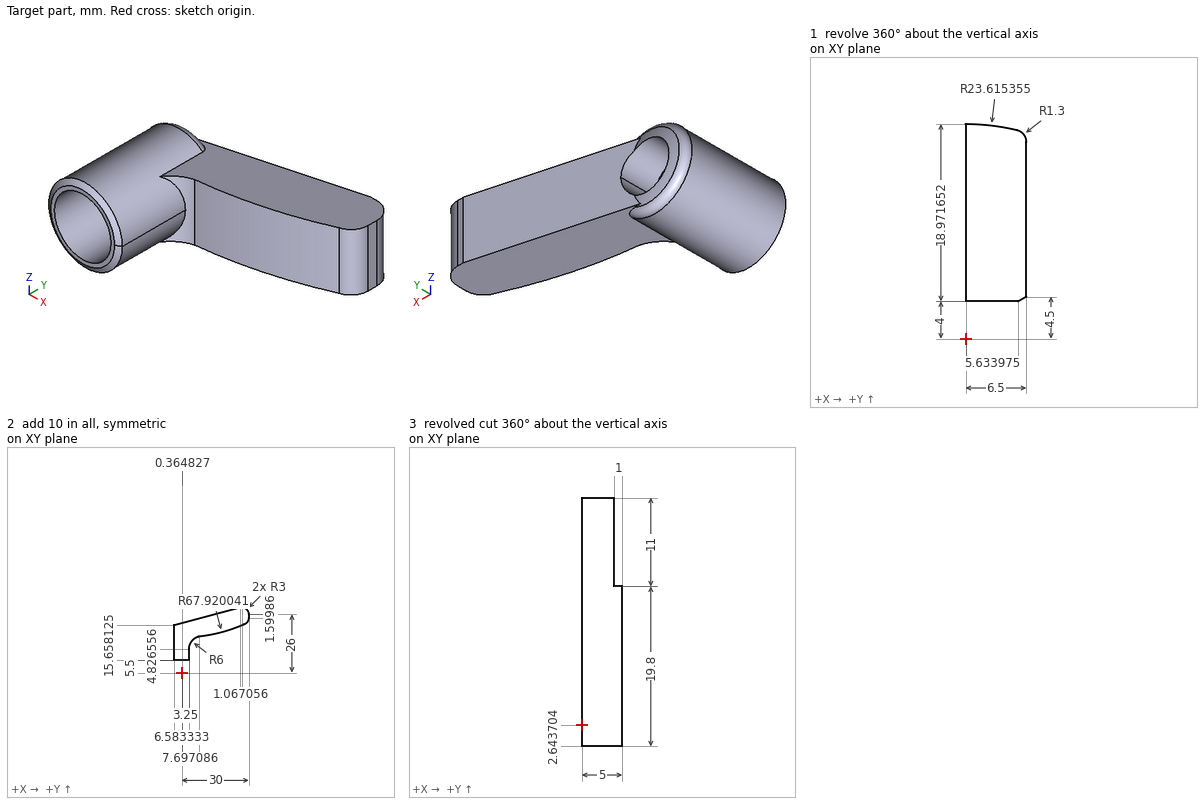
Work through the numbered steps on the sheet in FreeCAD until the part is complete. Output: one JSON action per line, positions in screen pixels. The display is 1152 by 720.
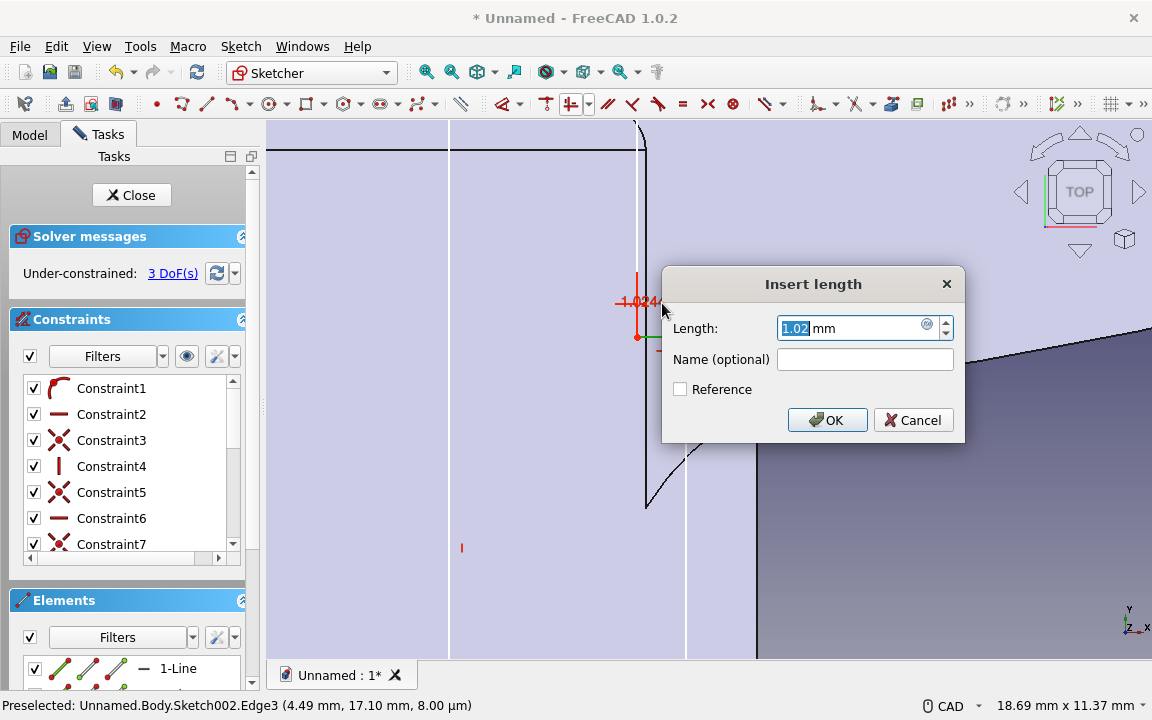
{"action": "type", "text": "1"}
{"action": "key", "text": "Return"}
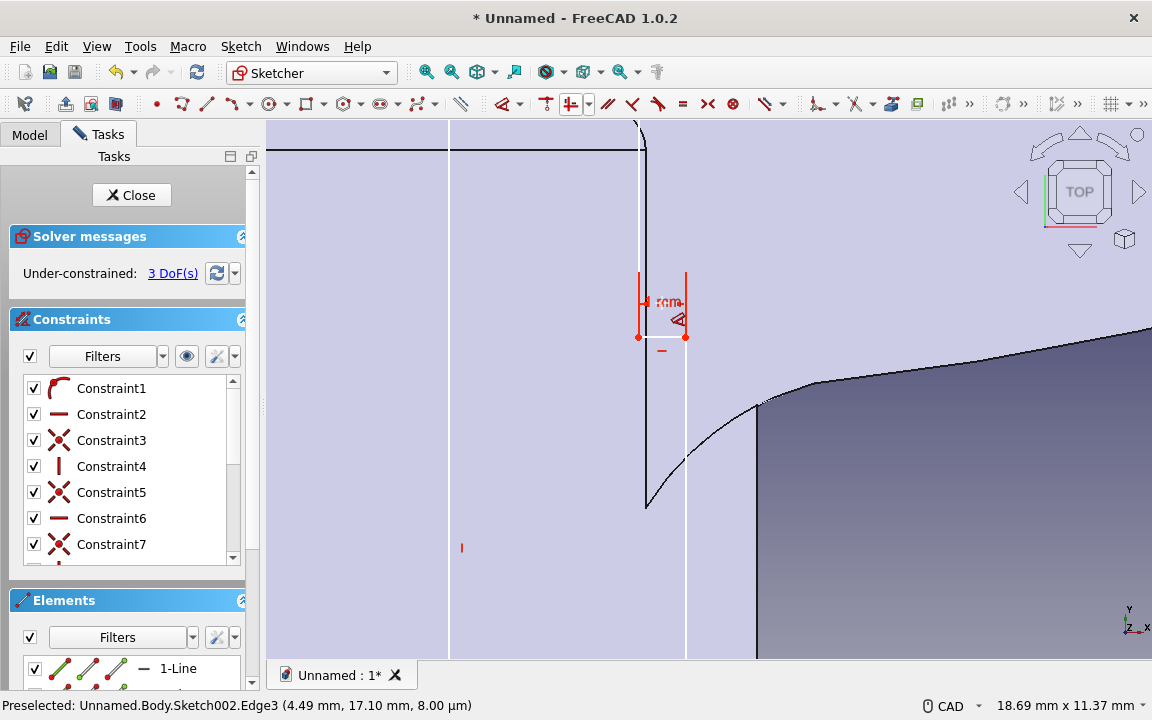
{"action": "scroll", "coordinate": [664, 339], "scroll_direction": "down", "scroll_amount": 7}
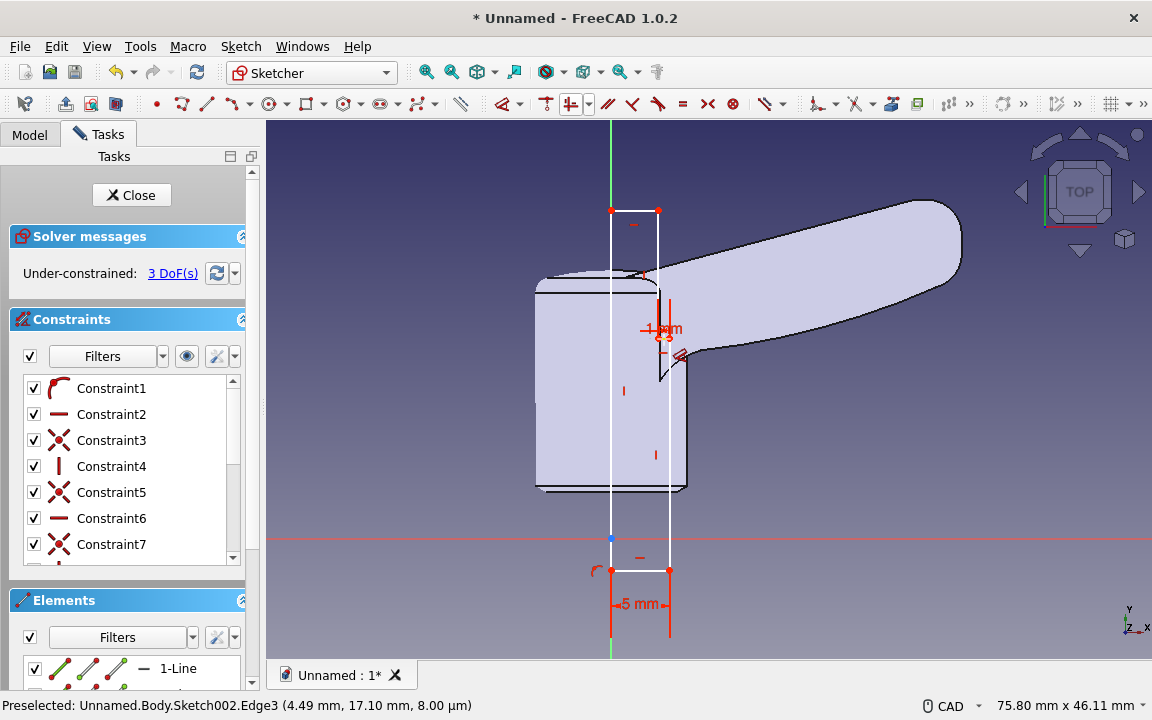
{"action": "left_click", "coordinate": [658, 300]}
{"action": "left_click", "coordinate": [692, 275]}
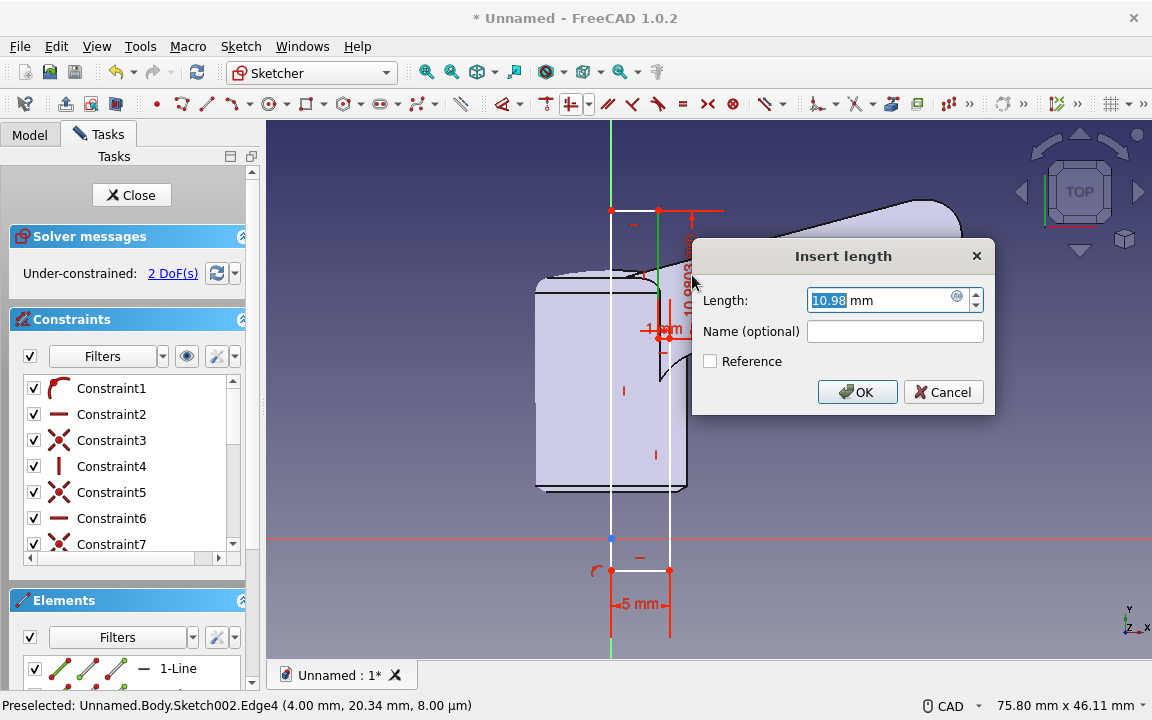
{"action": "type", "text": "11"}
{"action": "key", "text": "Return"}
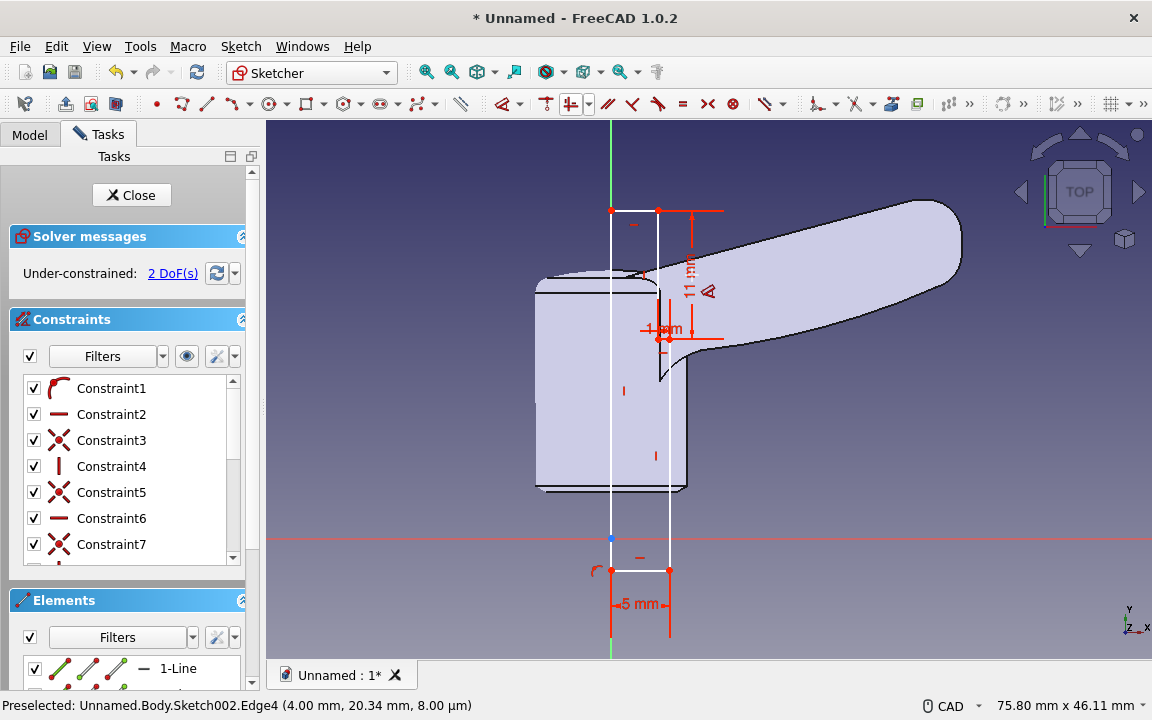
{"action": "left_click", "coordinate": [670, 501]}
{"action": "left_click", "coordinate": [704, 455]}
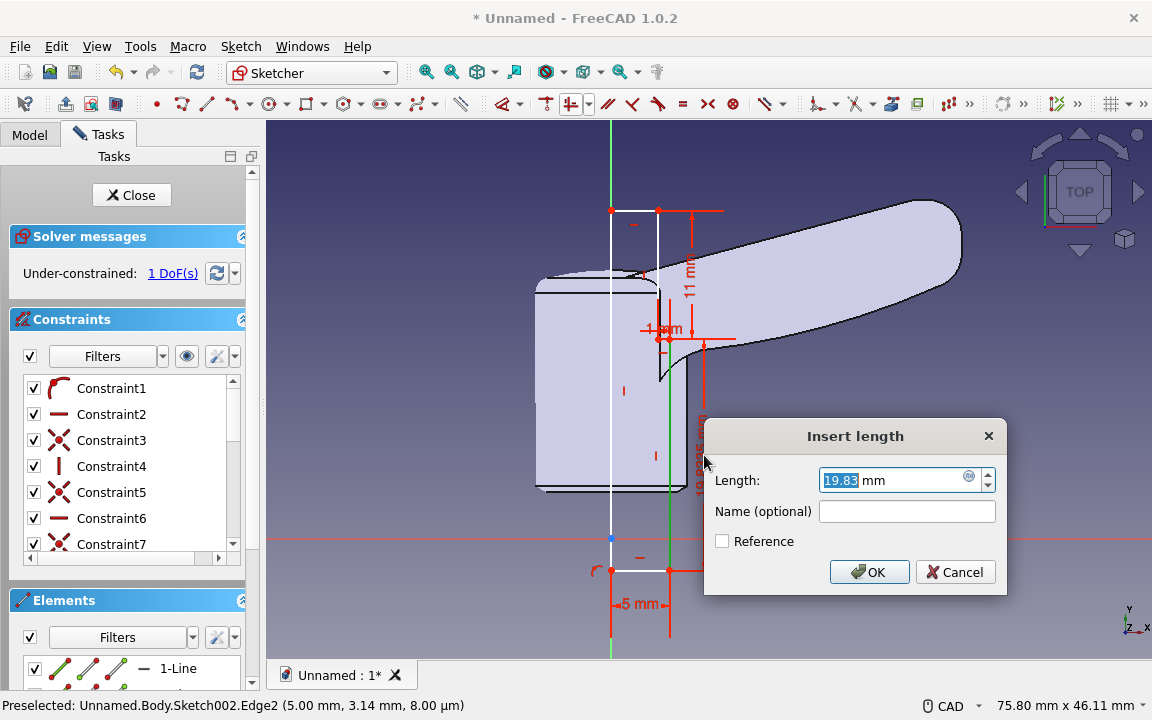
{"action": "type", "text": "19.8"}
{"action": "key", "text": "Return"}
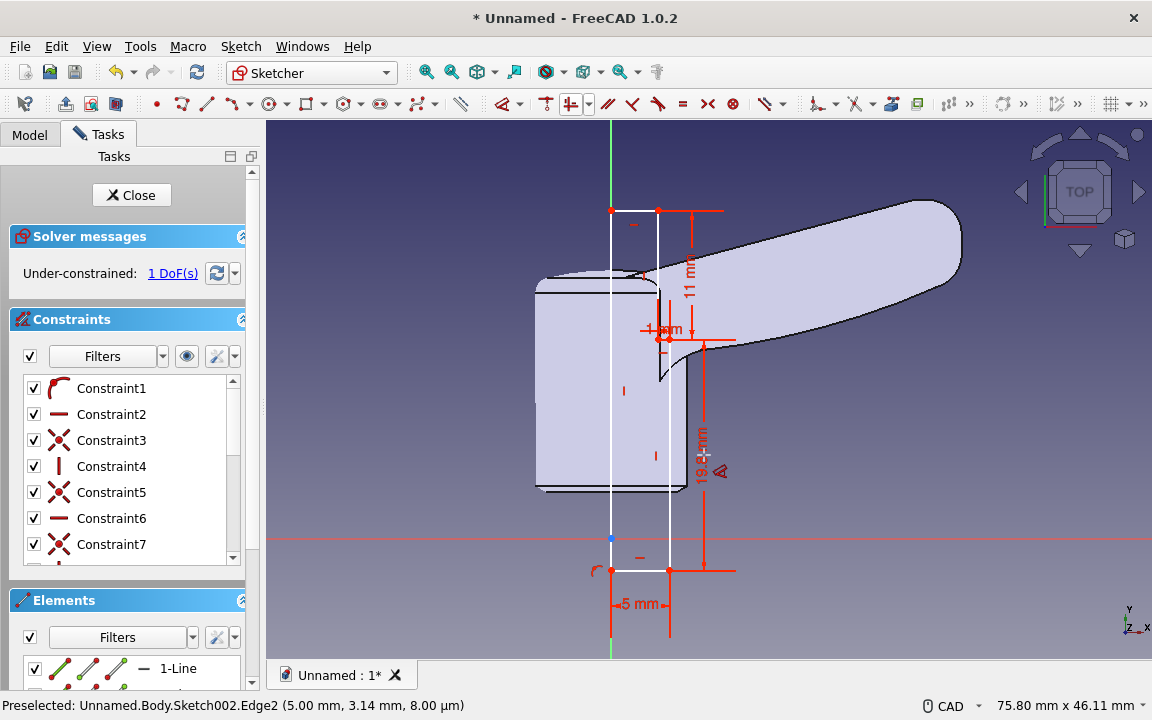
{"action": "scroll", "coordinate": [611, 571], "scroll_direction": "up", "scroll_amount": 2}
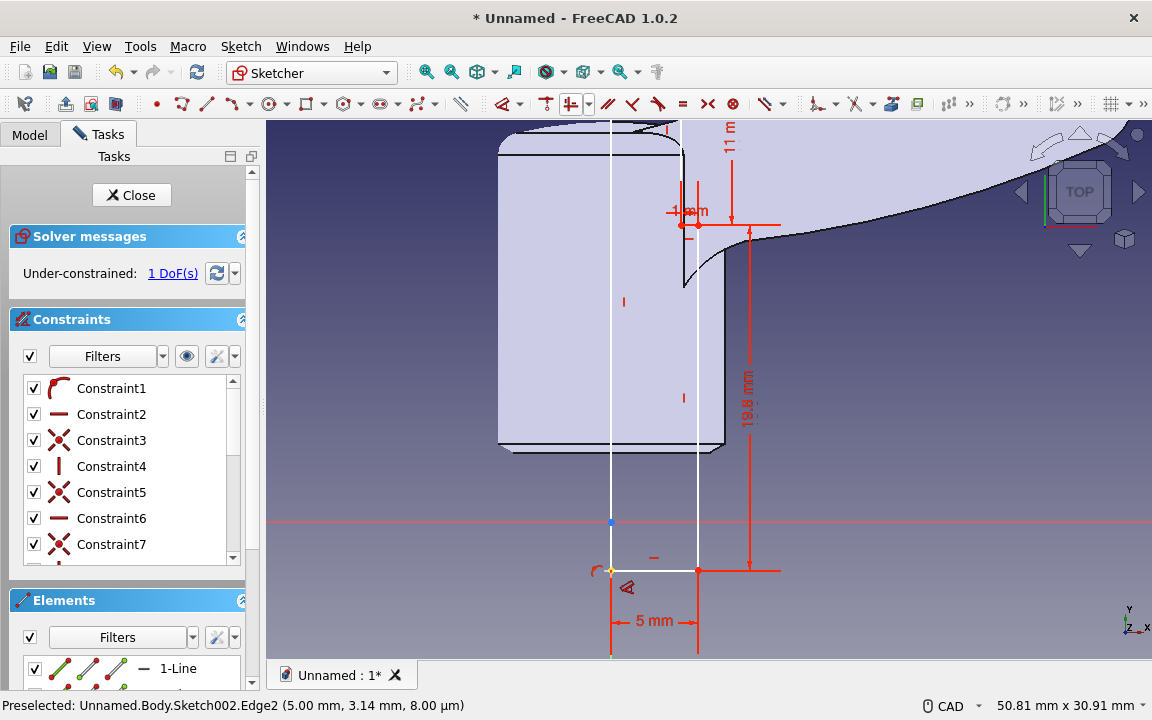
{"action": "left_click", "coordinate": [611, 571]}
{"action": "left_click", "coordinate": [577, 546]}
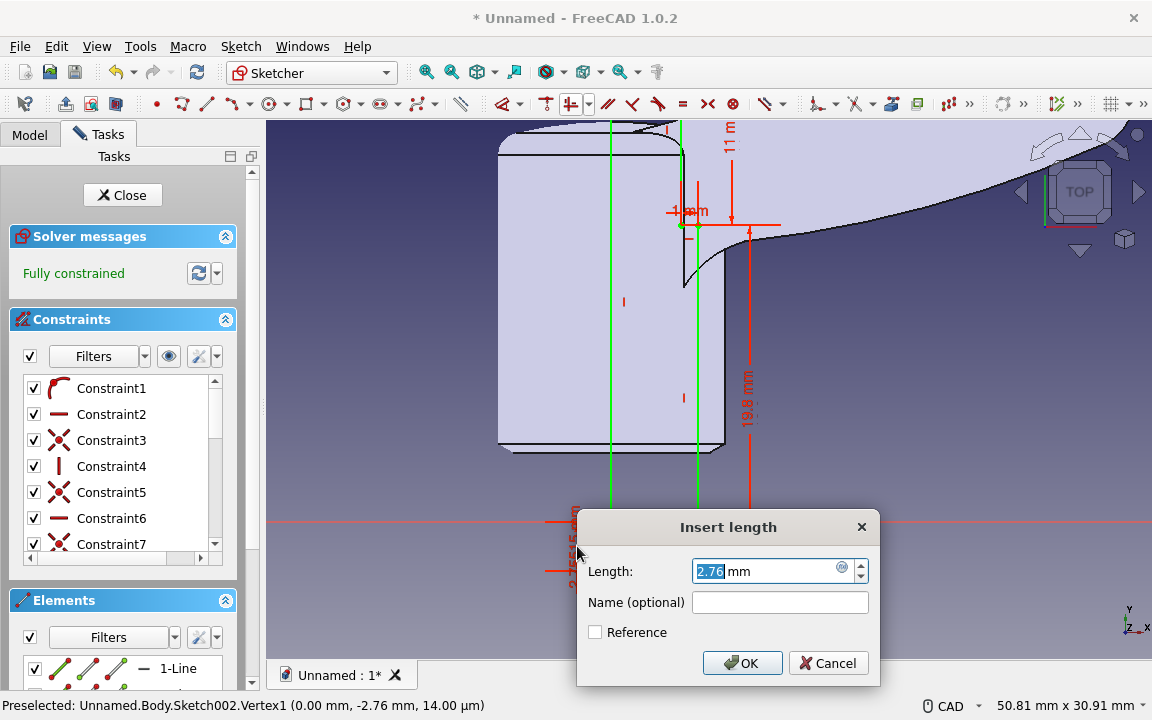
{"action": "type", "text": "2.643704"}
{"action": "key", "text": "Return"}
{"action": "key", "text": "Escape"}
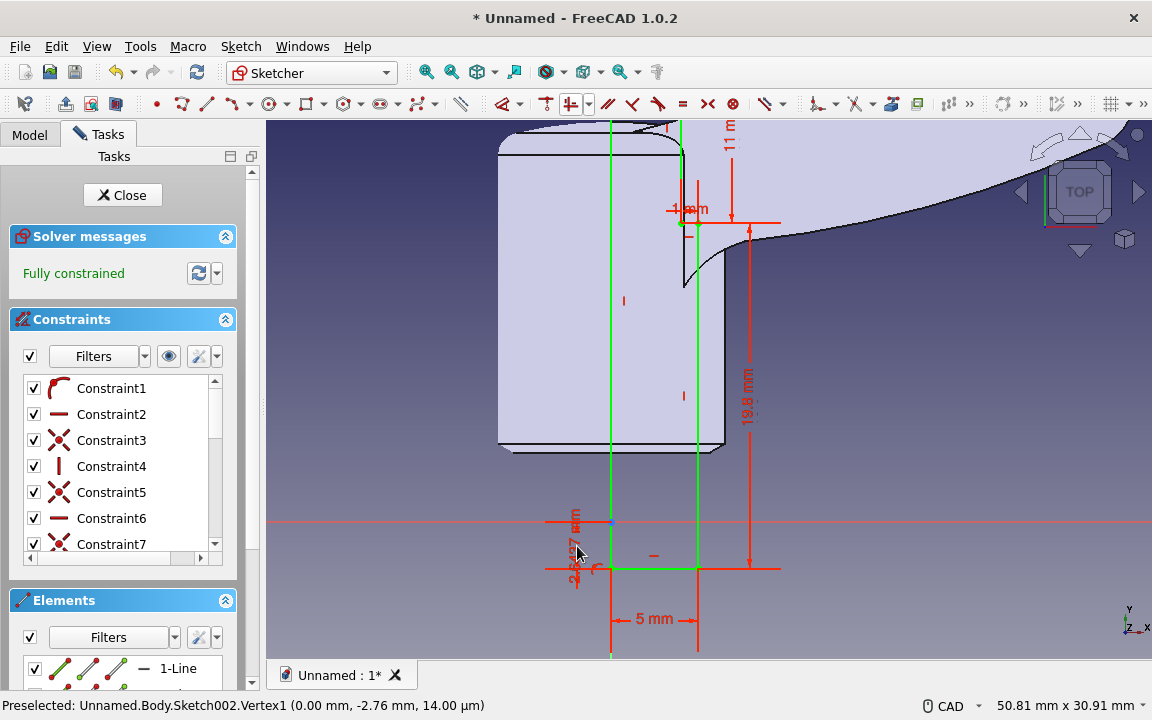
{"action": "left_click", "coordinate": [123, 195]}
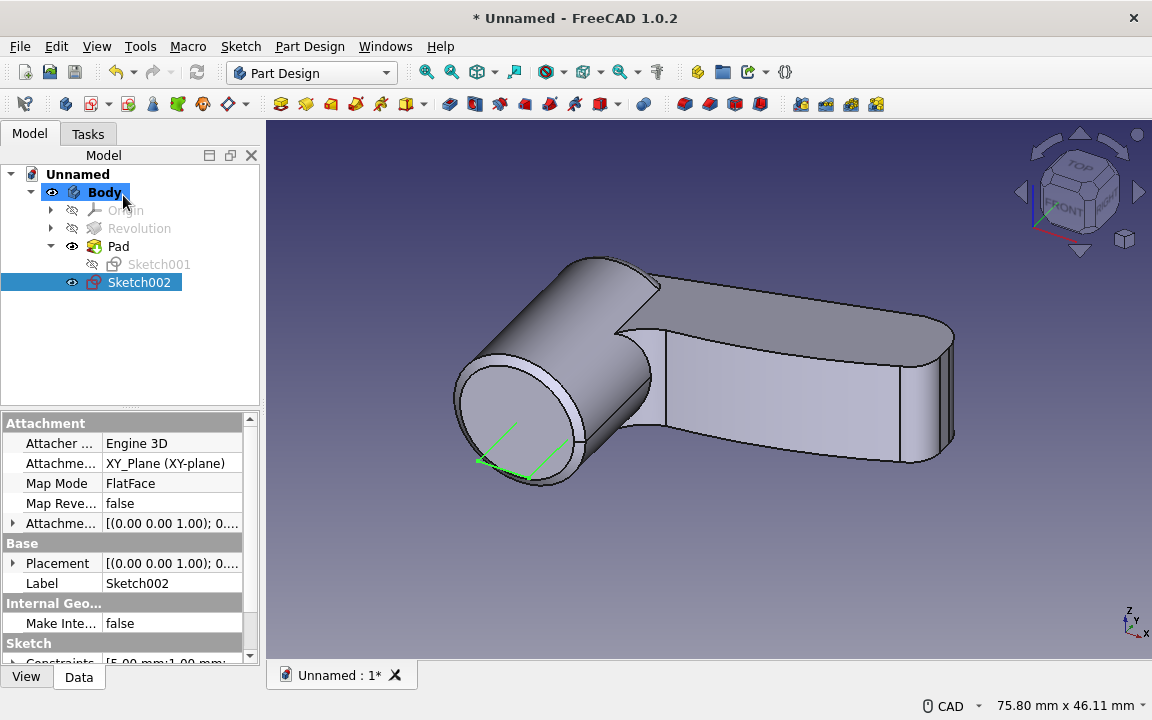
{"action": "left_click", "coordinate": [500, 104]}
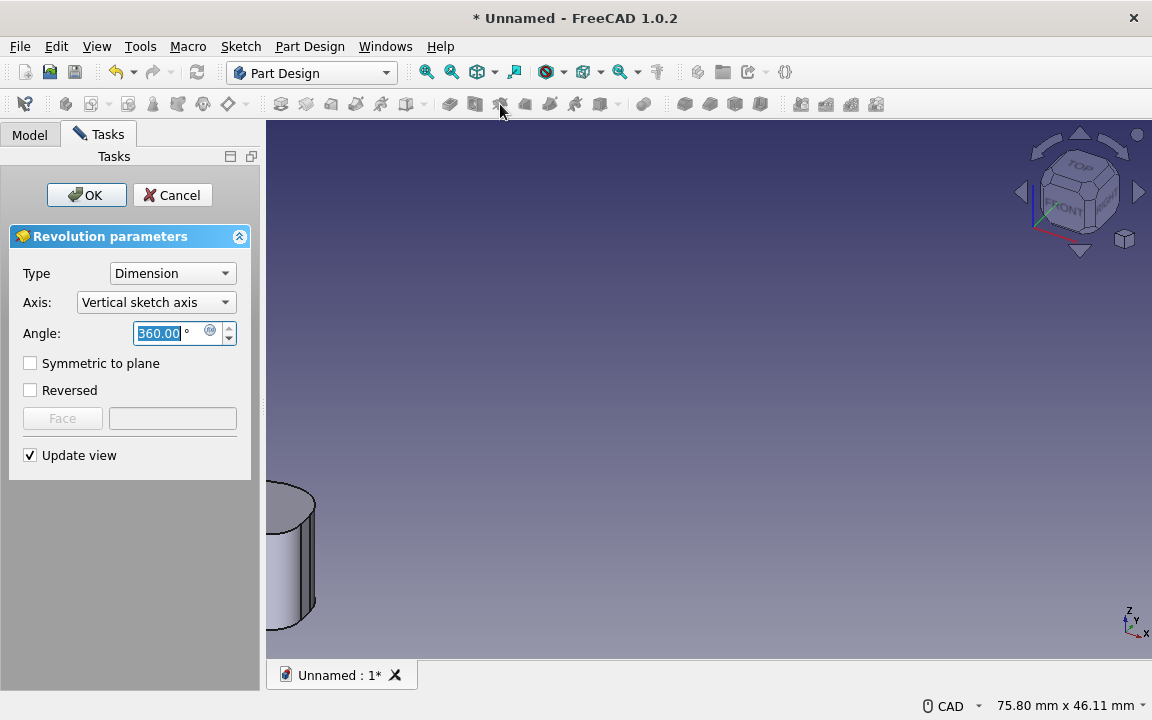
{"action": "left_click", "coordinate": [87, 195]}